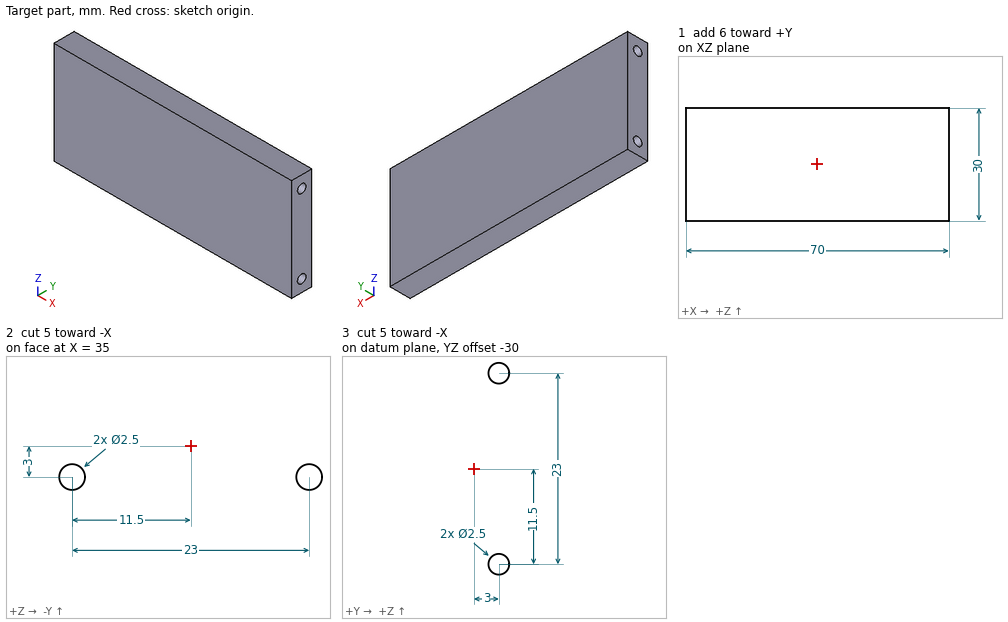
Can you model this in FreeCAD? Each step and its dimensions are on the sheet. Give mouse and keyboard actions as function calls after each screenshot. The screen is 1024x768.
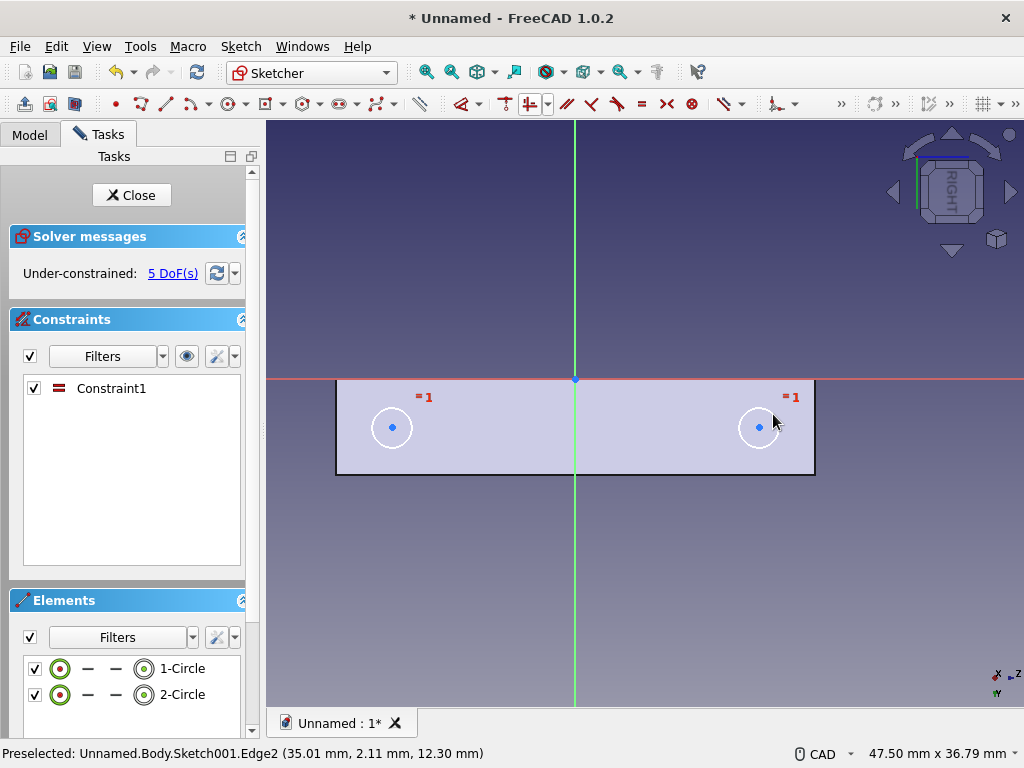
click(392, 428)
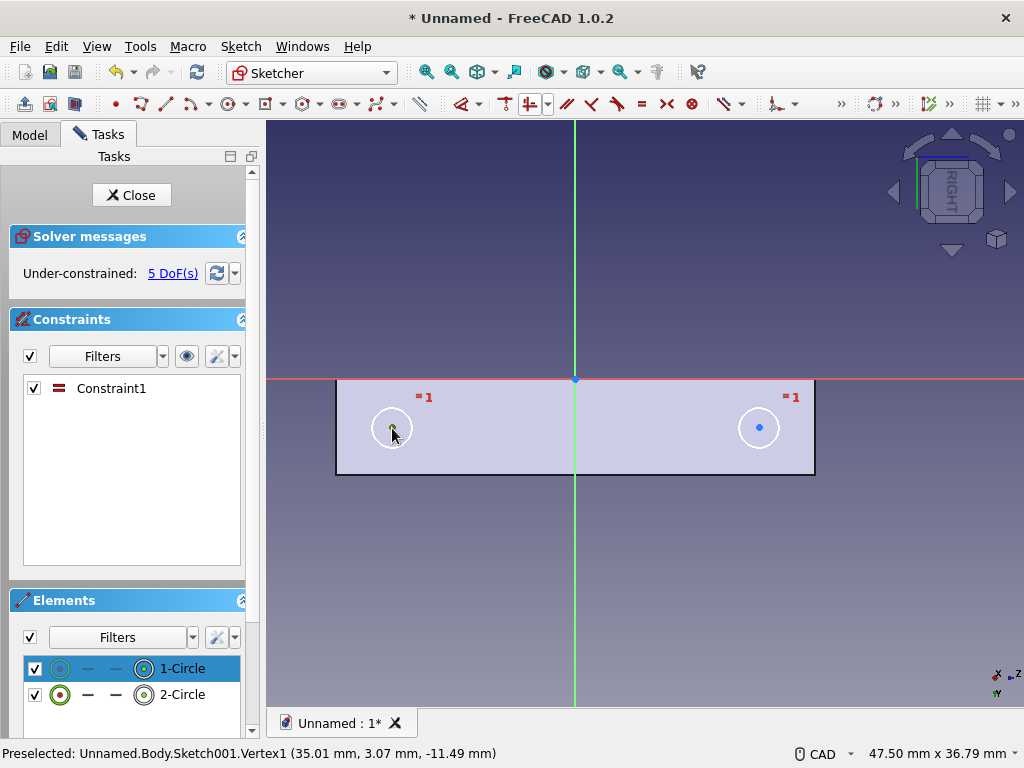
click(759, 428)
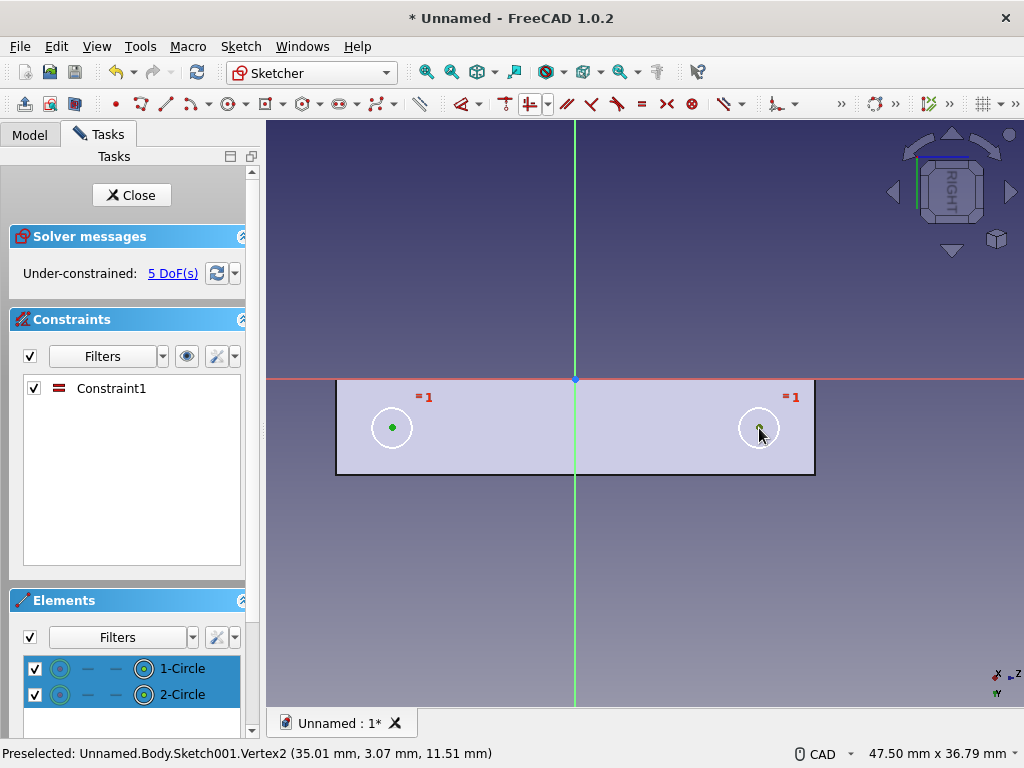
key(h)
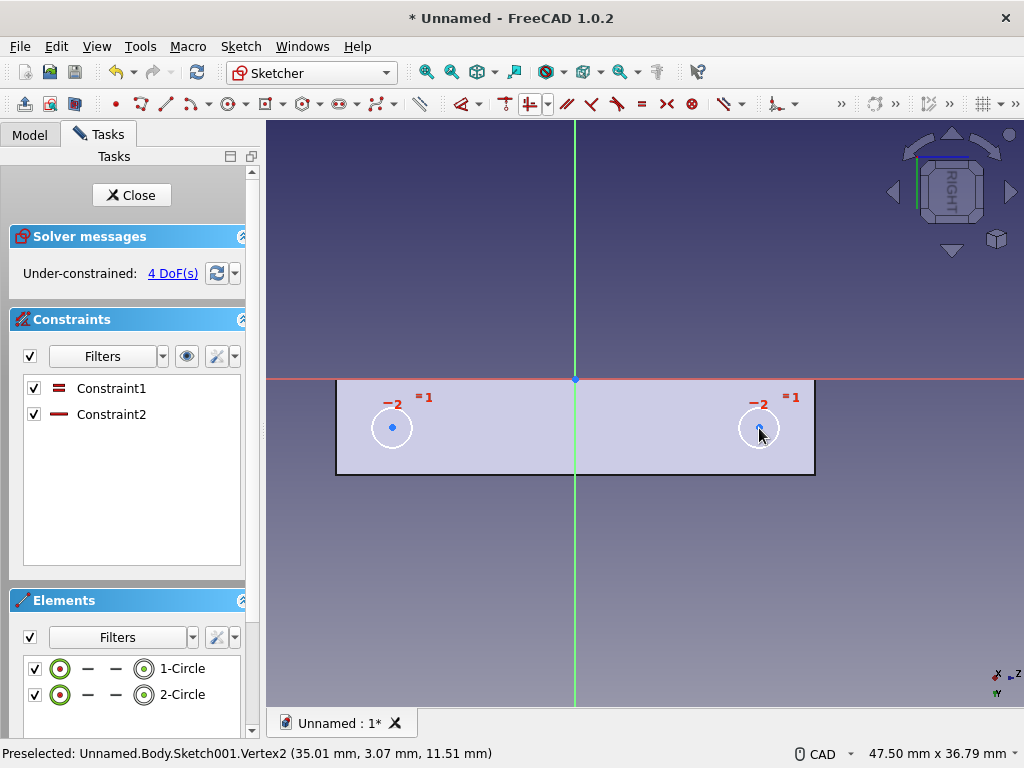
click(460, 104)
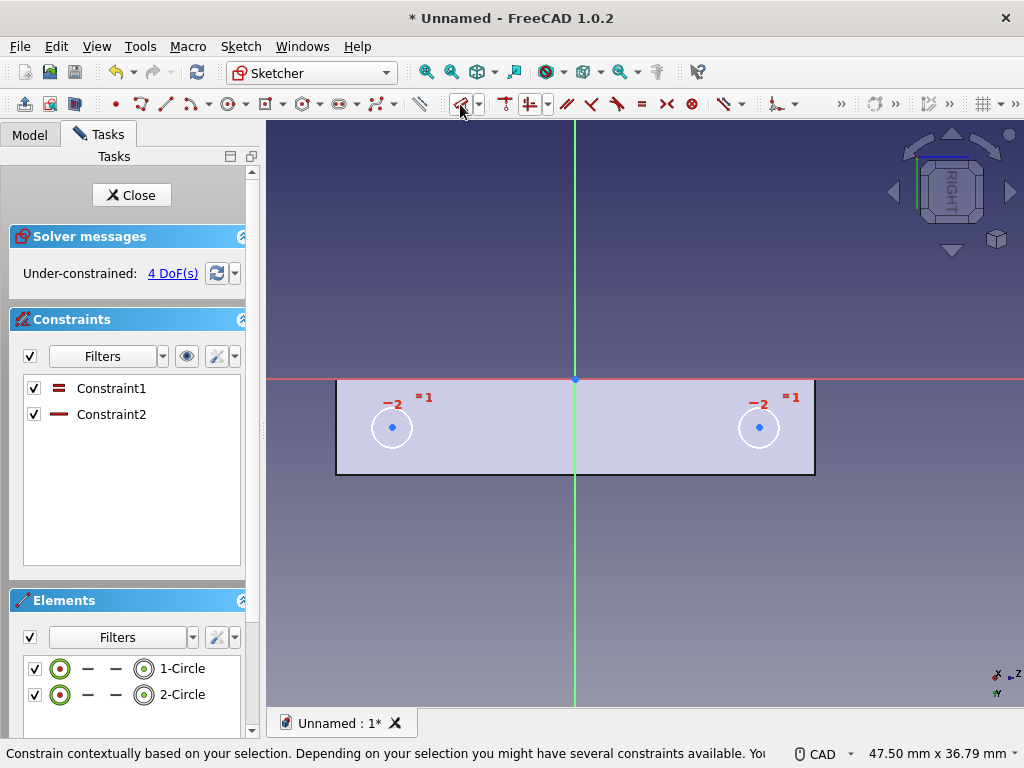
click(406, 414)
click(442, 413)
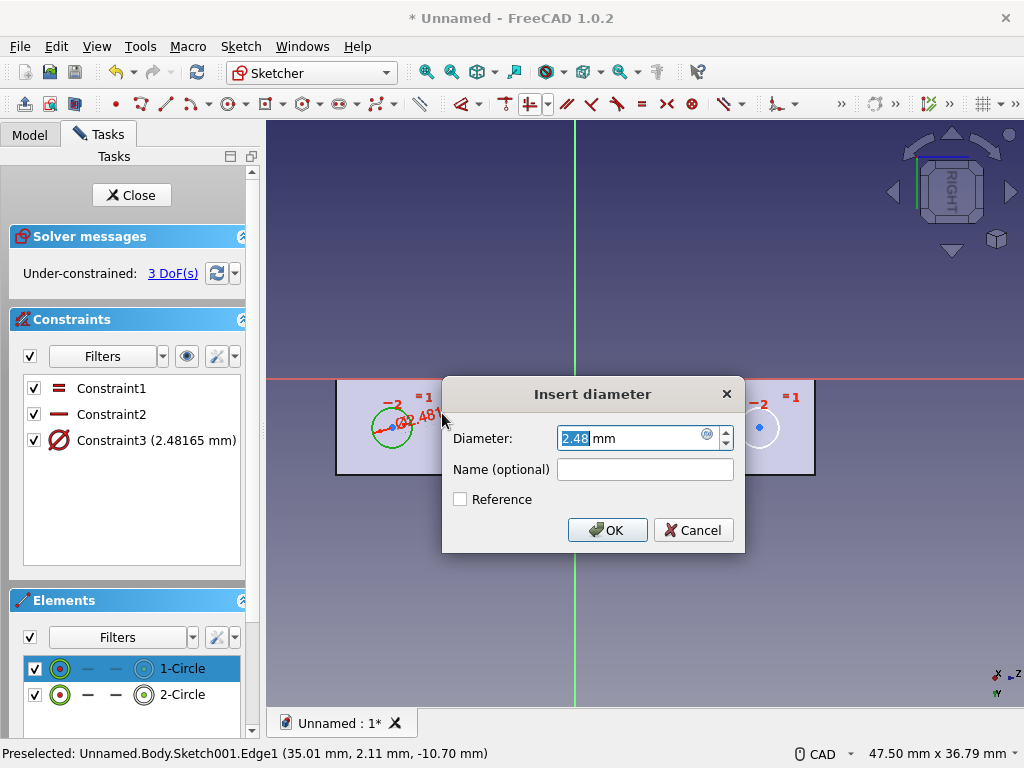
text(2.5)
key(Return)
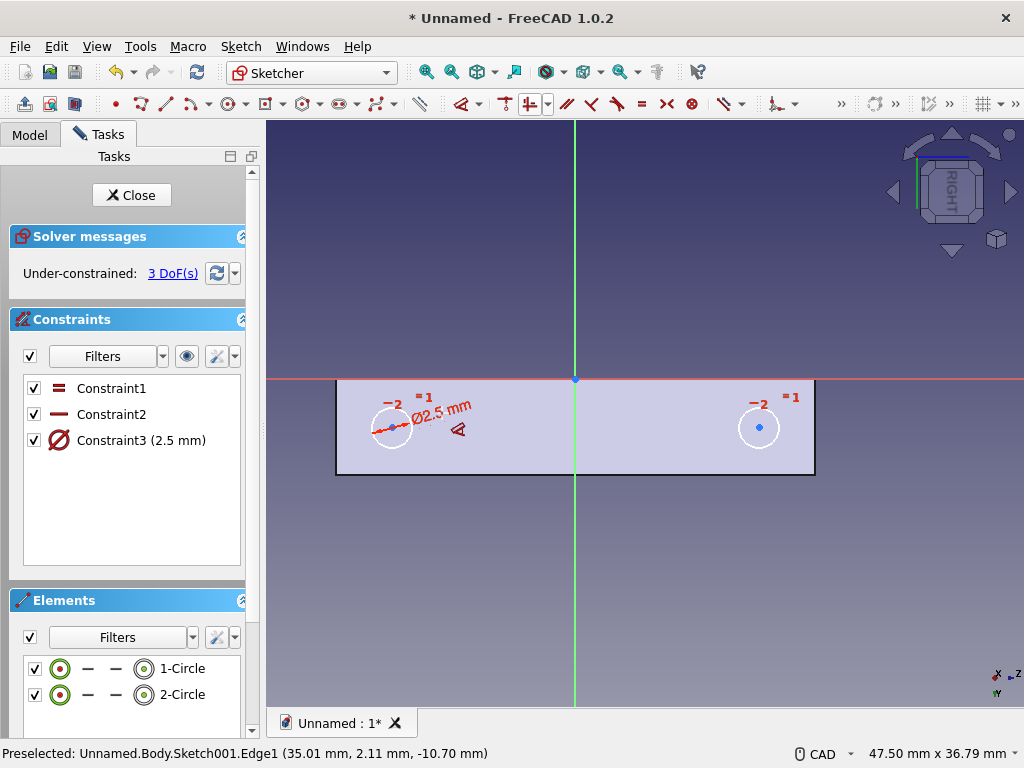
click(392, 428)
click(358, 404)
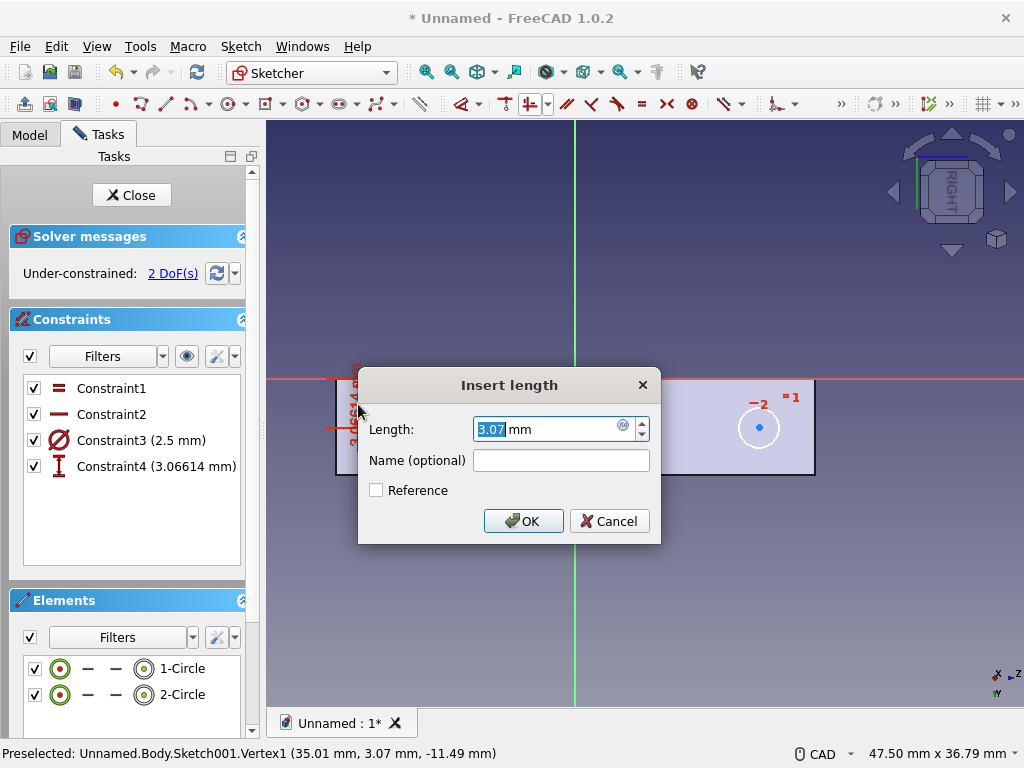
text(3)
key(Return)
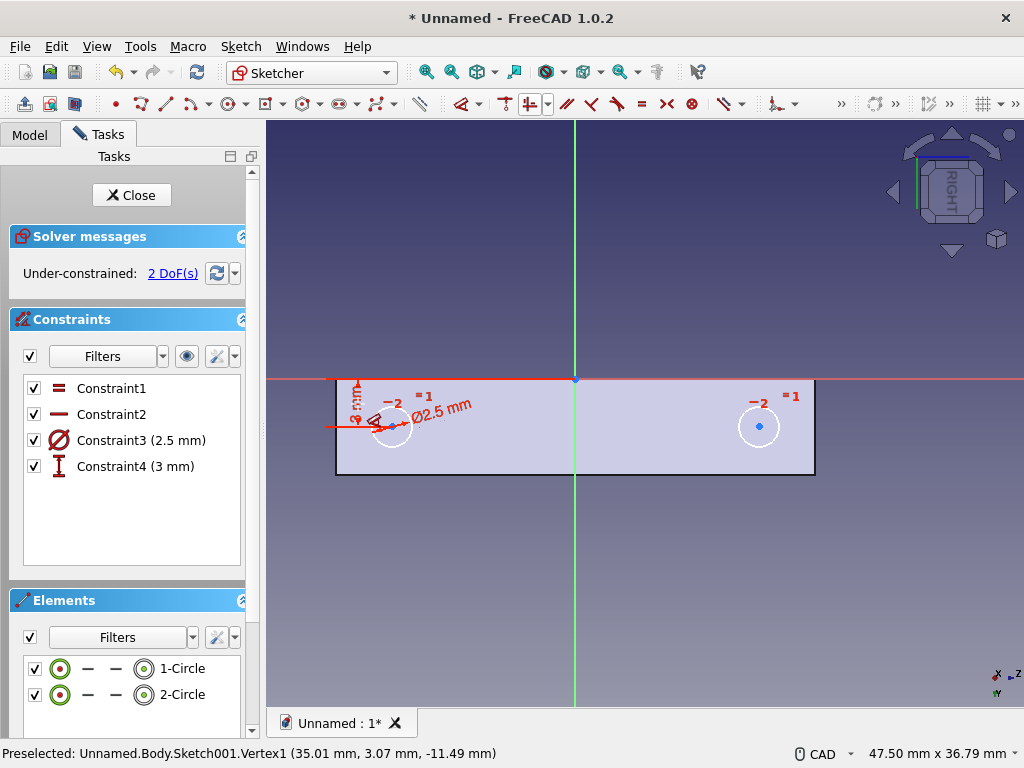
click(392, 427)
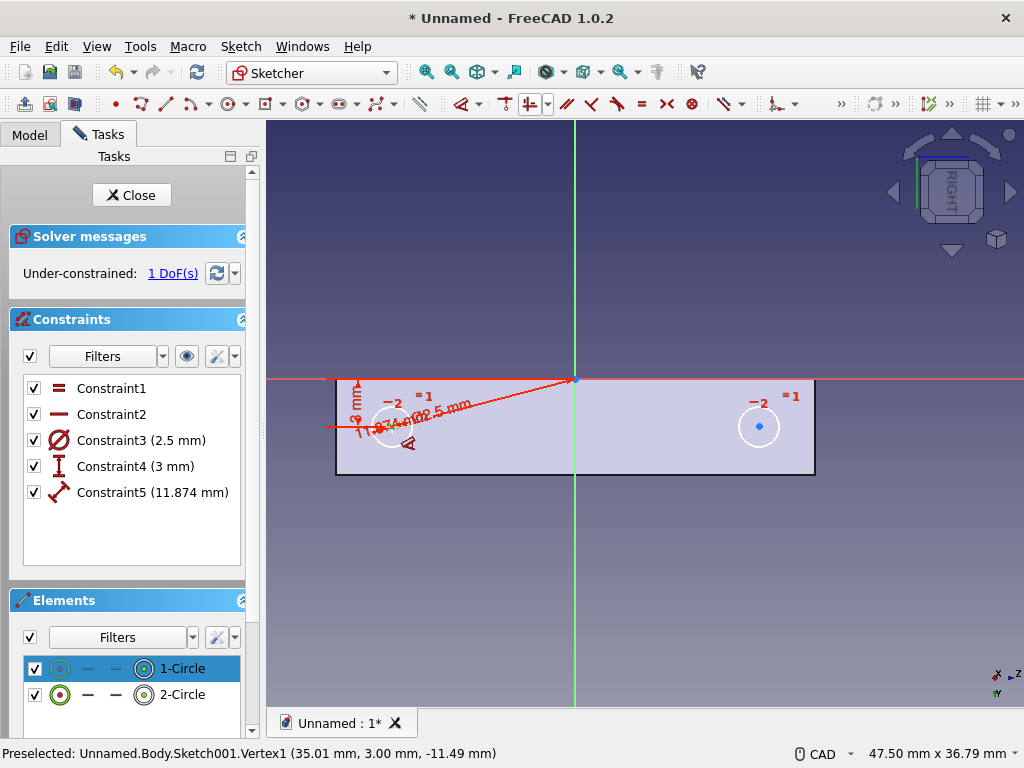
click(759, 427)
click(491, 461)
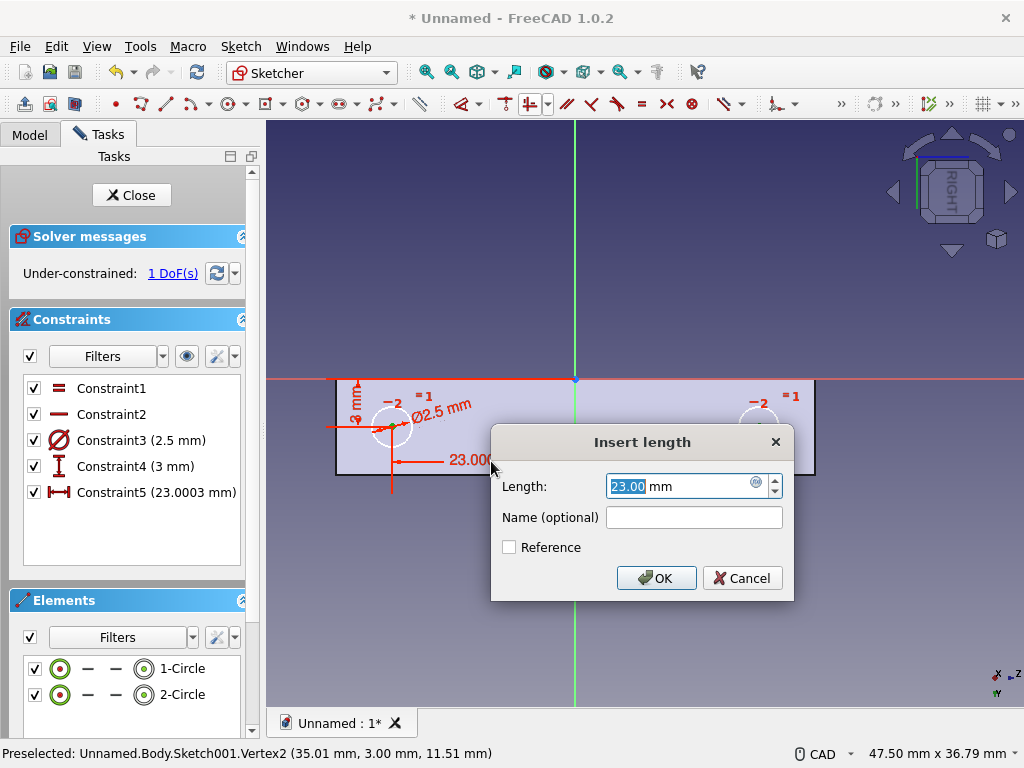
text(23)
key(Return)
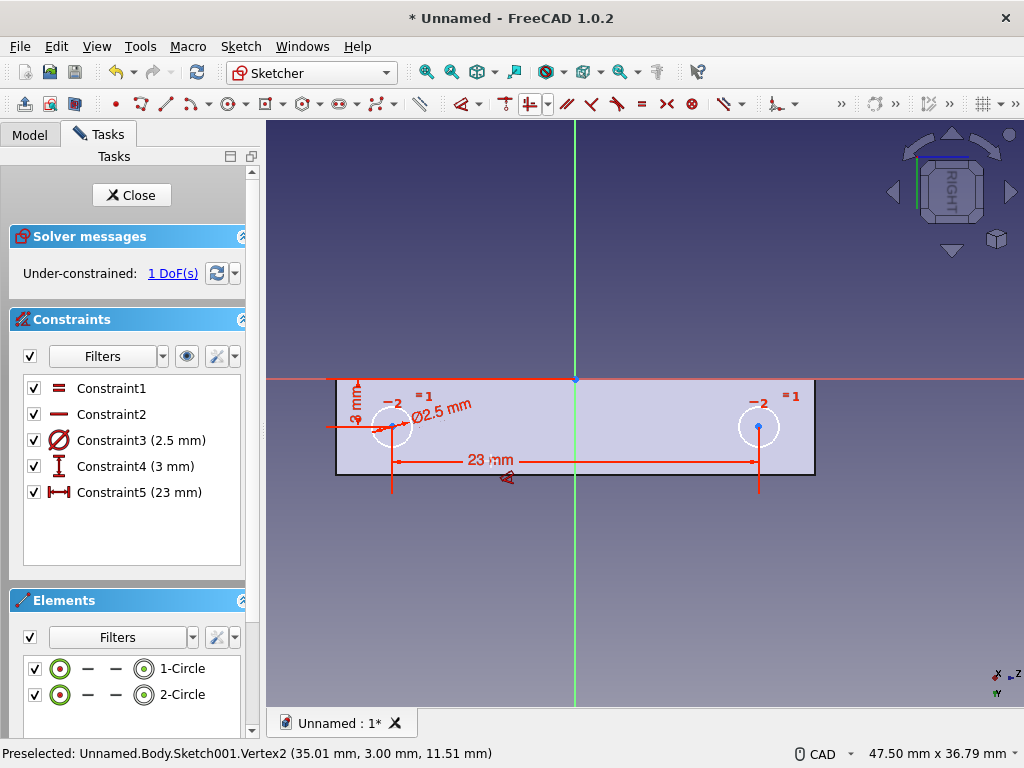
click(392, 427)
click(484, 345)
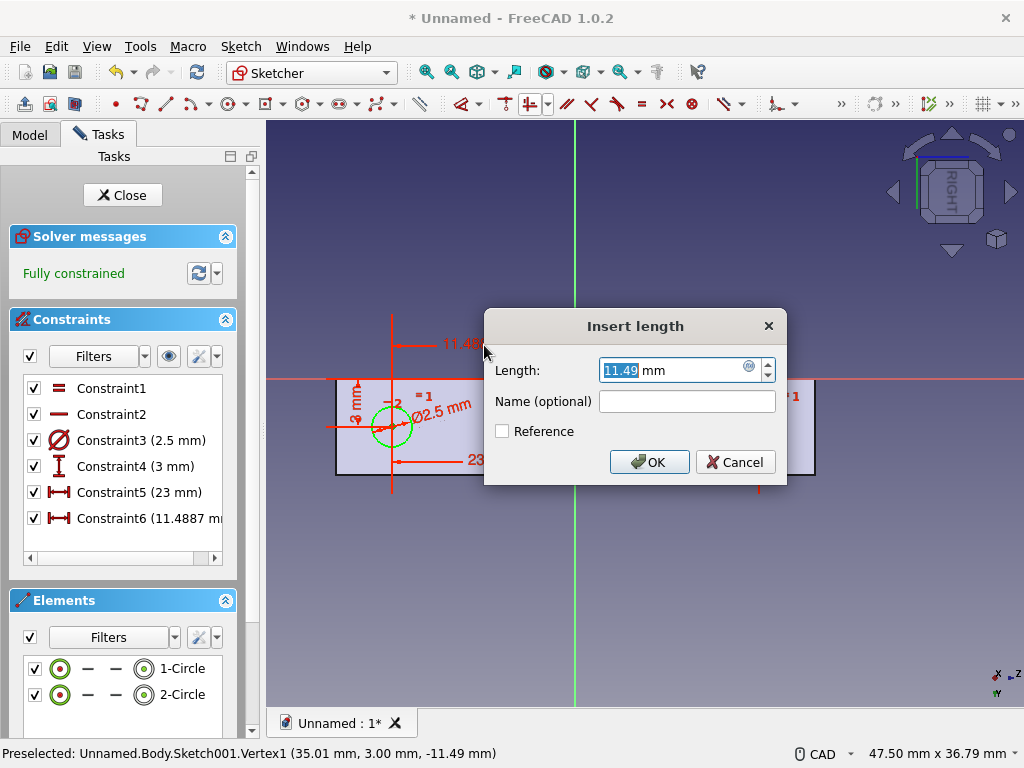
text(11.5)
key(Return)
key(Escape)